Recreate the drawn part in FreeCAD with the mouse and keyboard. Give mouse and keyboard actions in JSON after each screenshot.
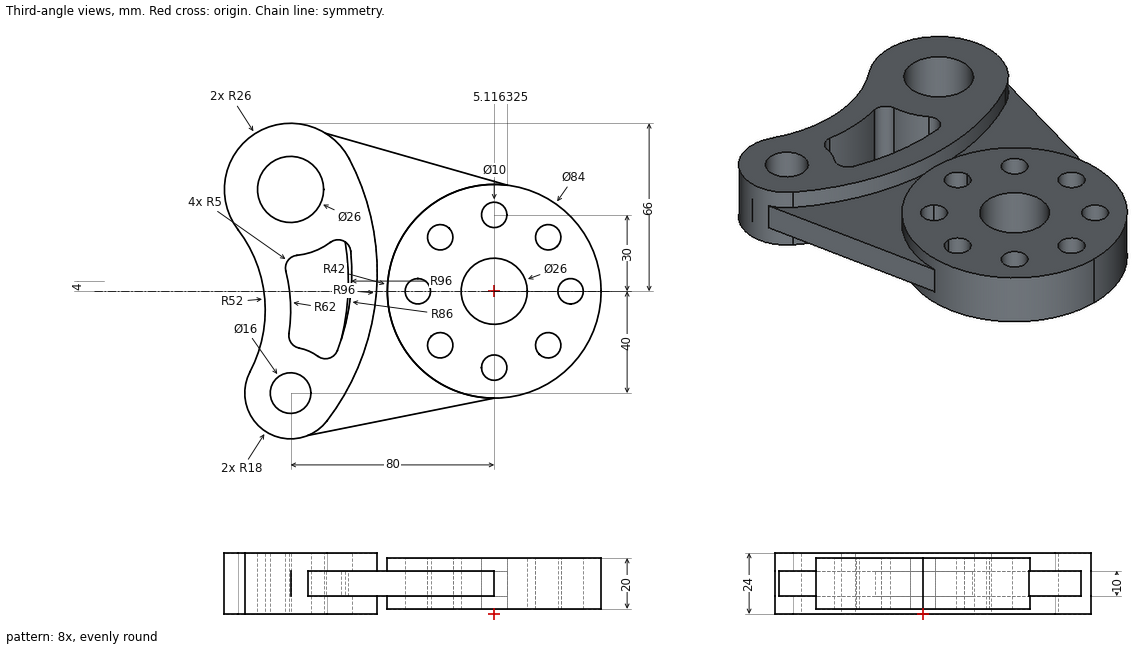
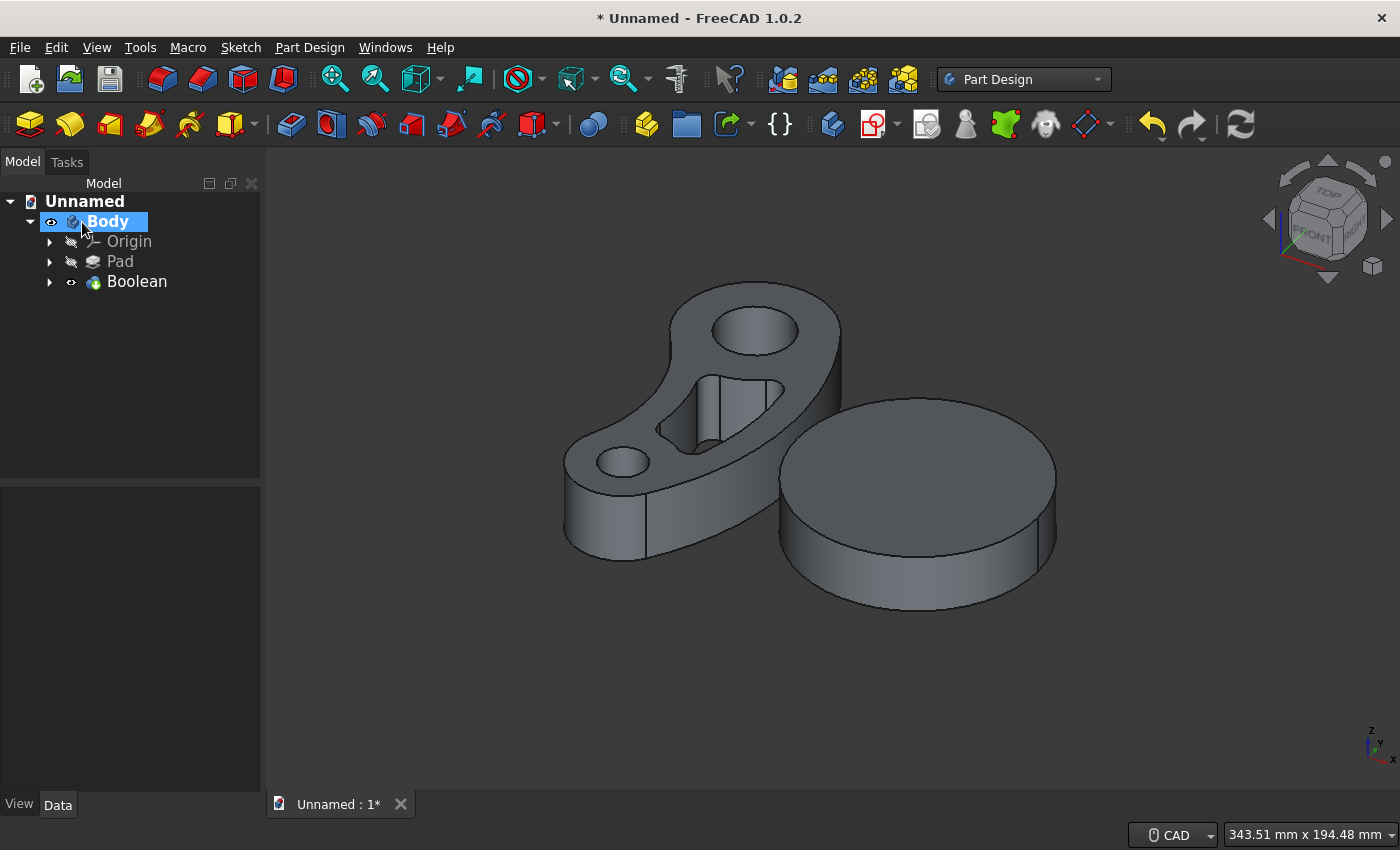
{"action": "left_click", "coordinate": [50, 242]}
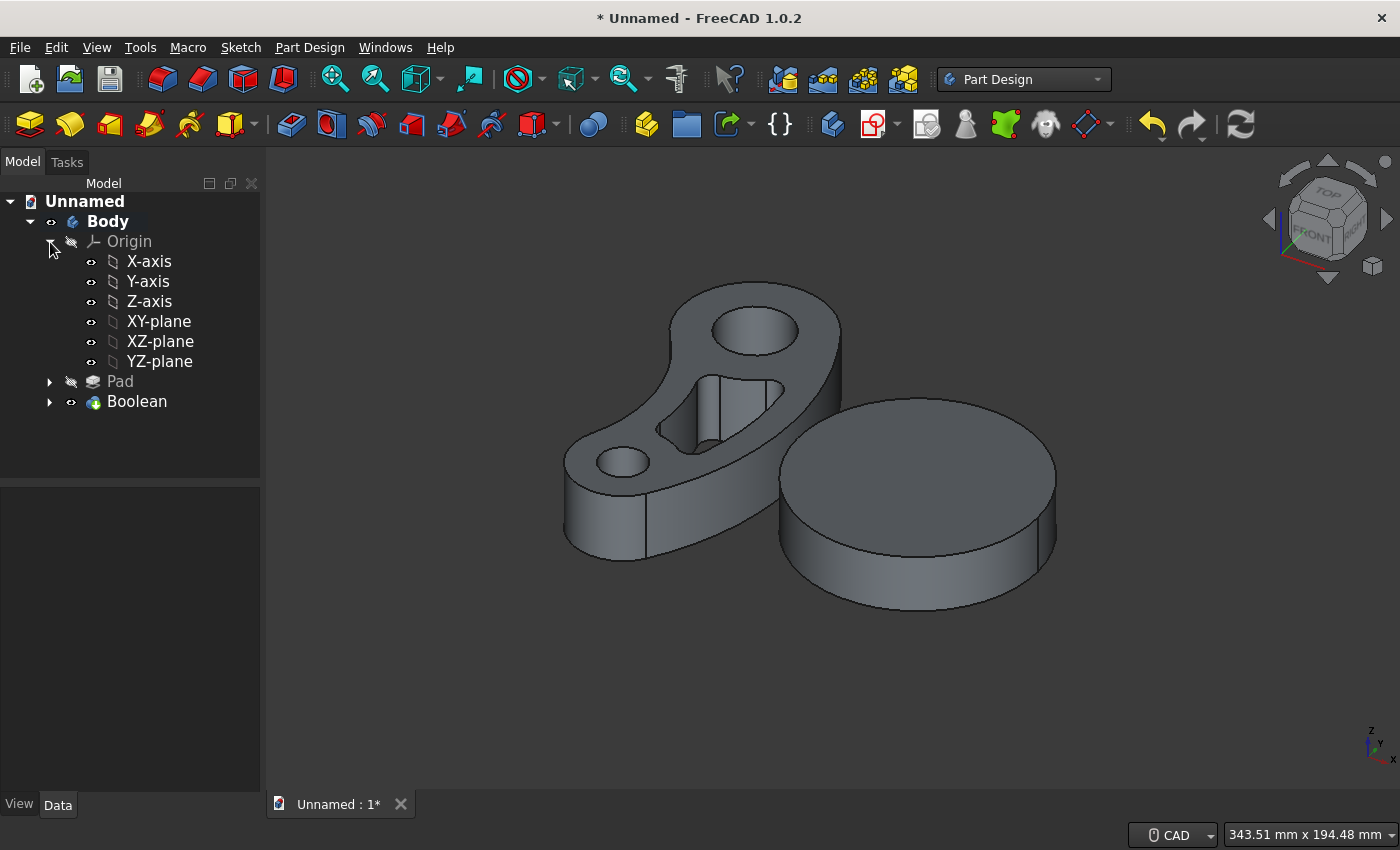
{"action": "left_click", "coordinate": [136, 322]}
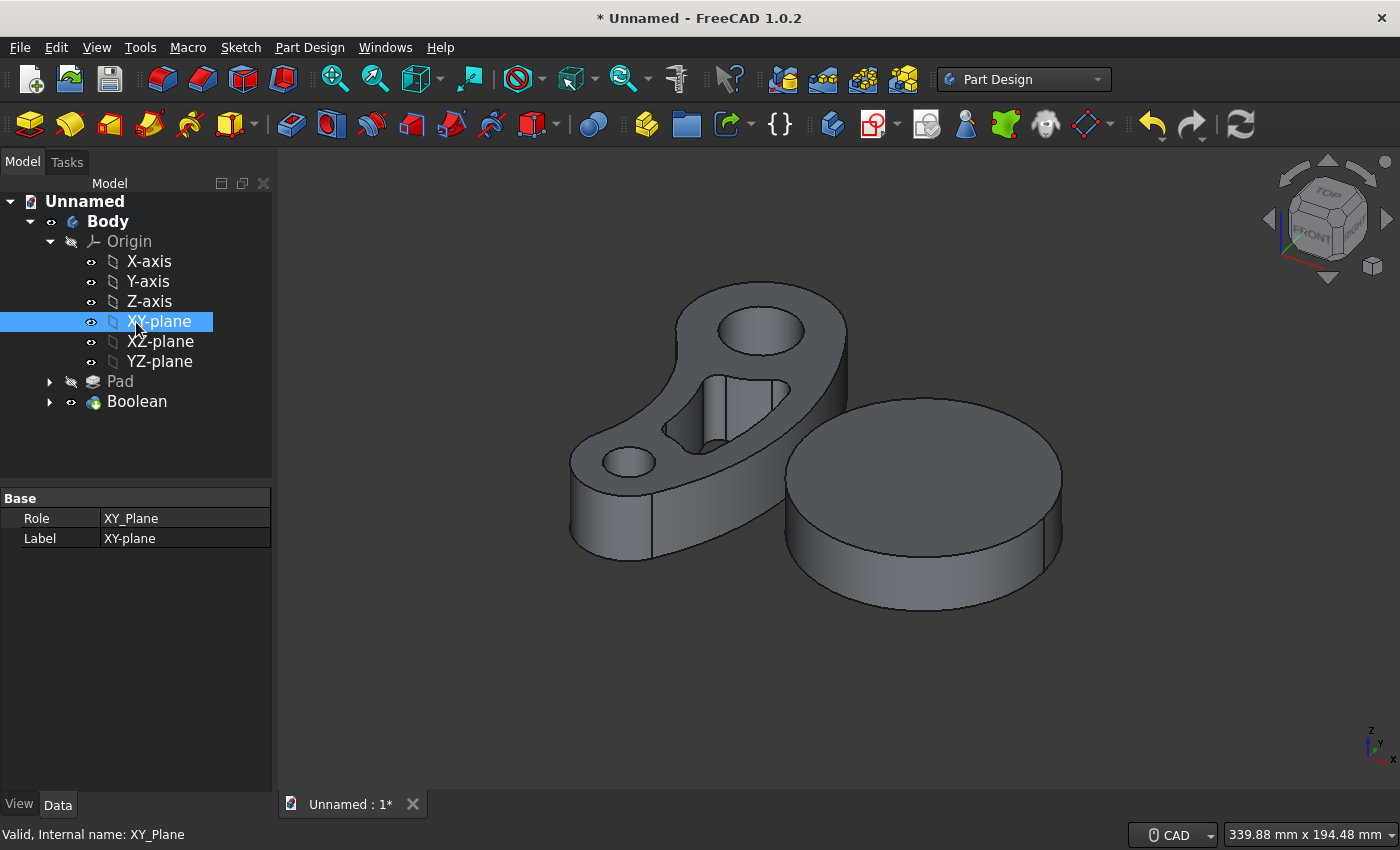
{"action": "left_click", "coordinate": [1086, 124]}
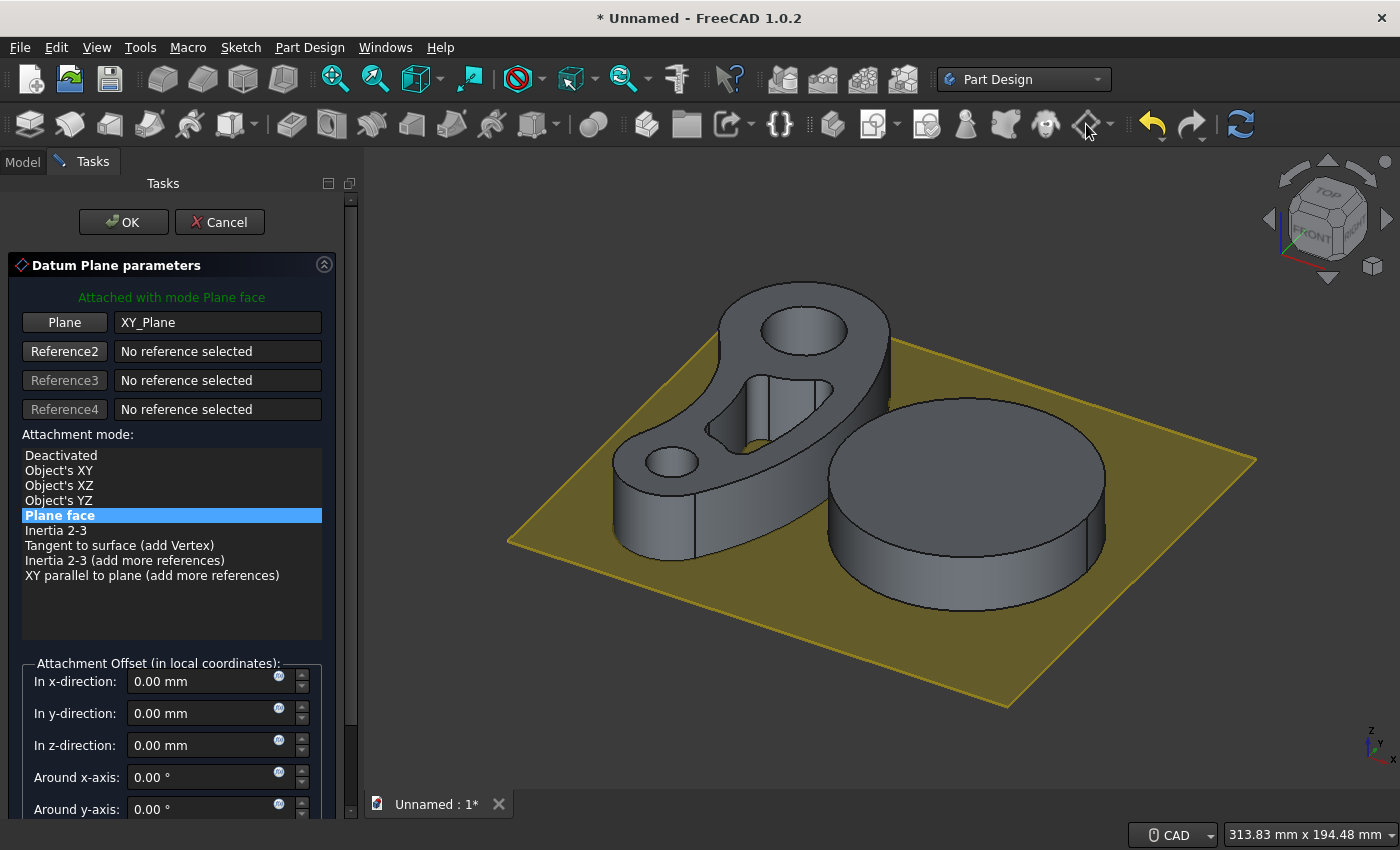
{"action": "triple_click", "coordinate": [210, 745]}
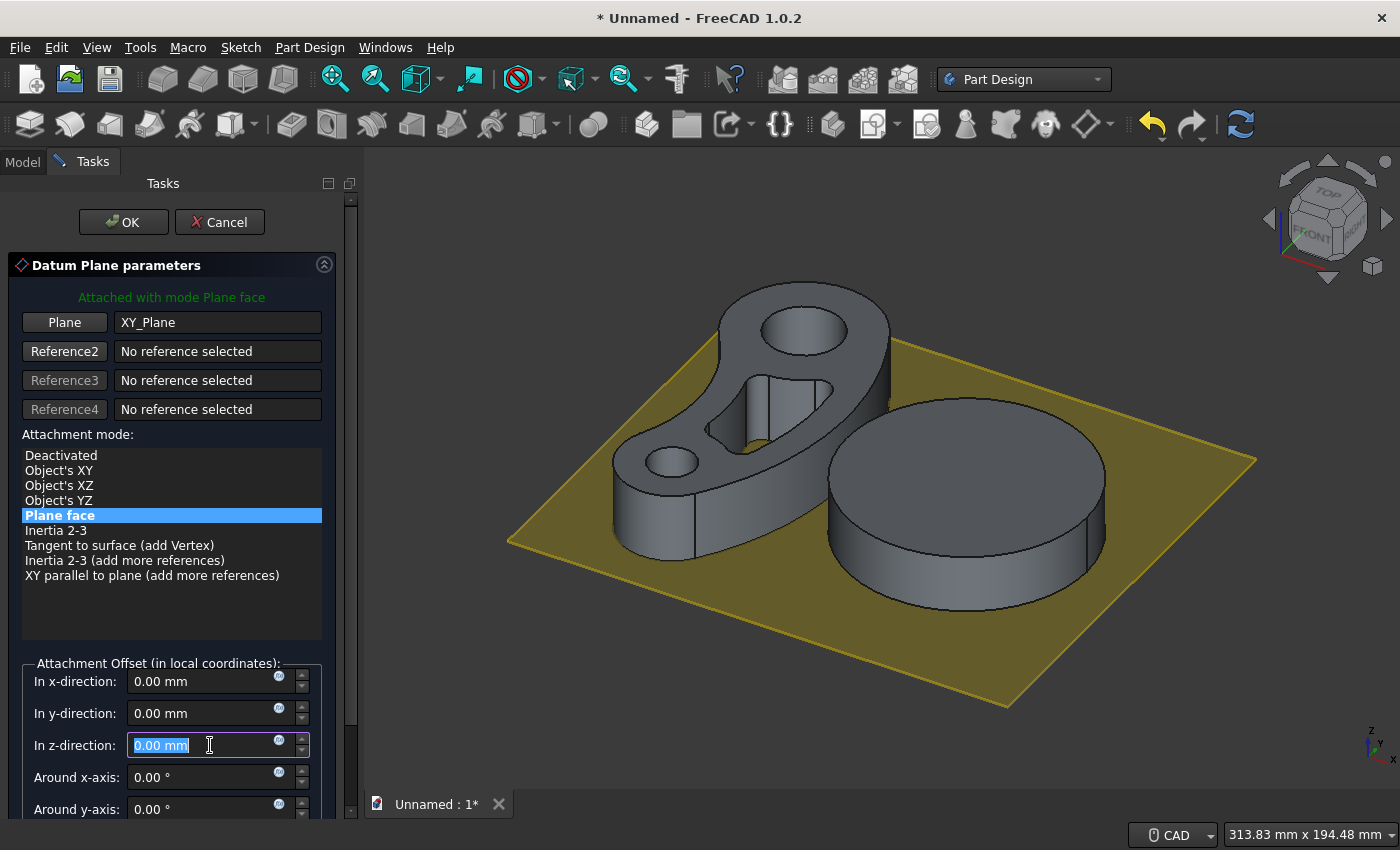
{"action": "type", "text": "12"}
{"action": "key", "text": "Tab"}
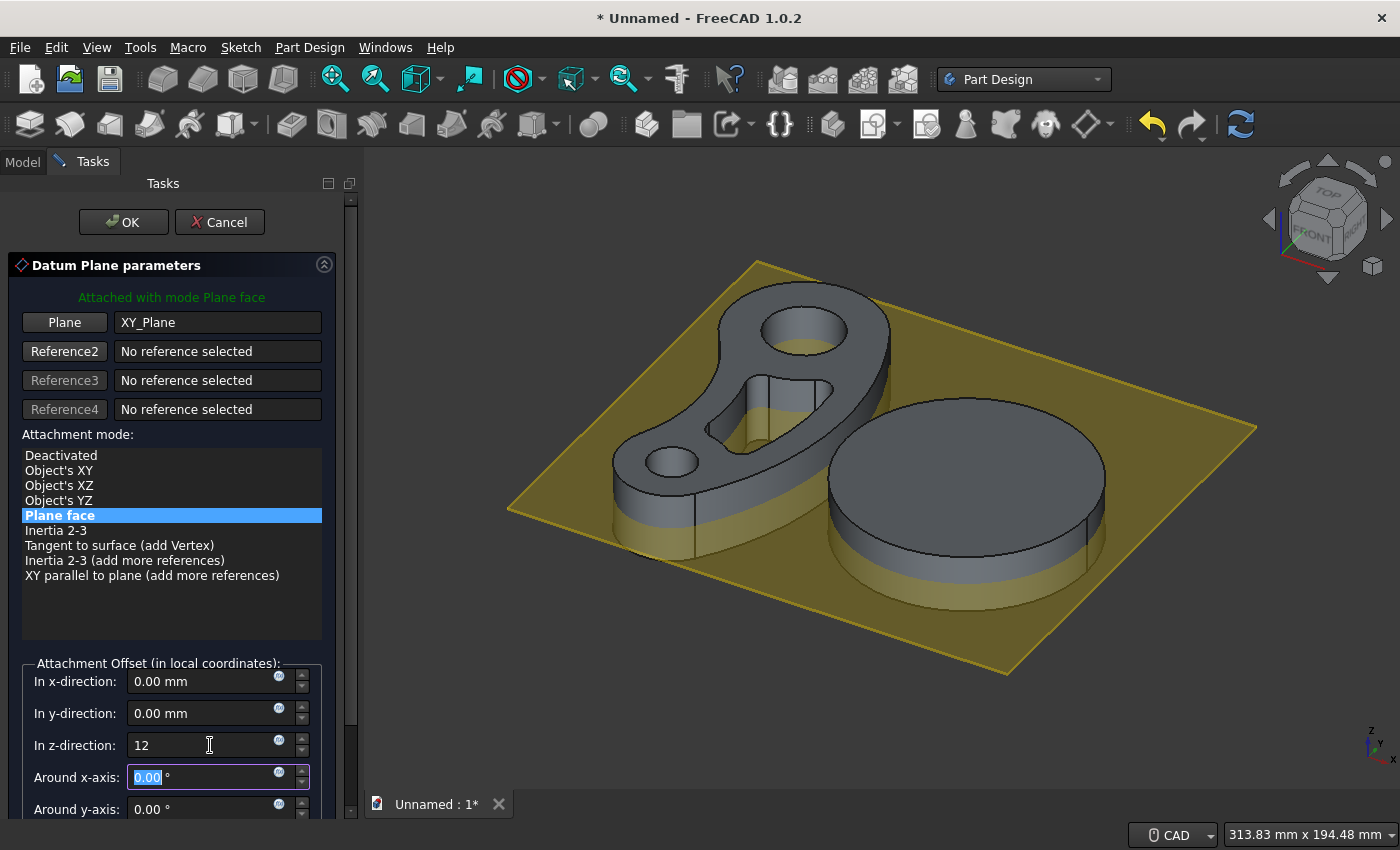
{"action": "left_click", "coordinate": [124, 222]}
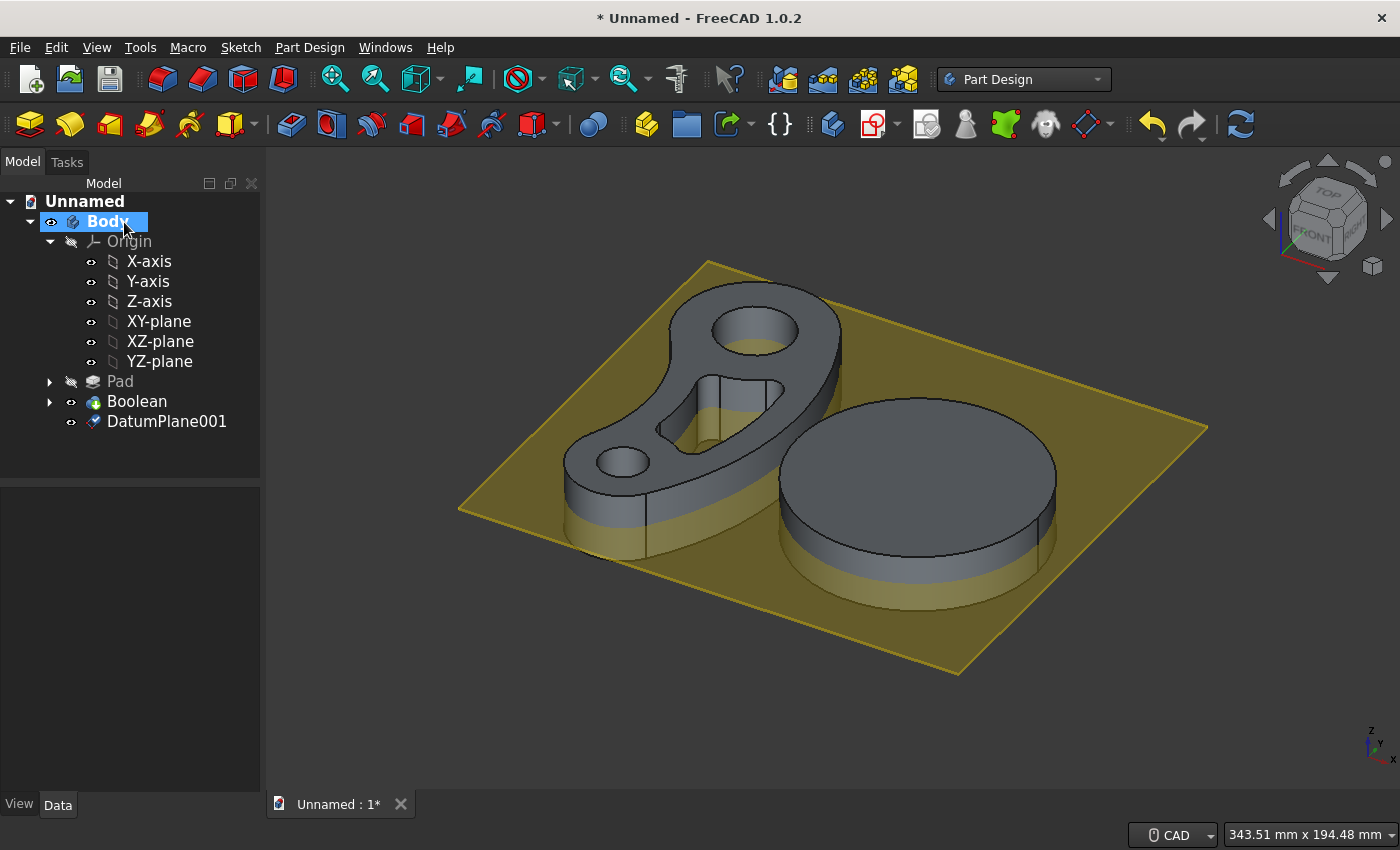
{"action": "left_click", "coordinate": [116, 422]}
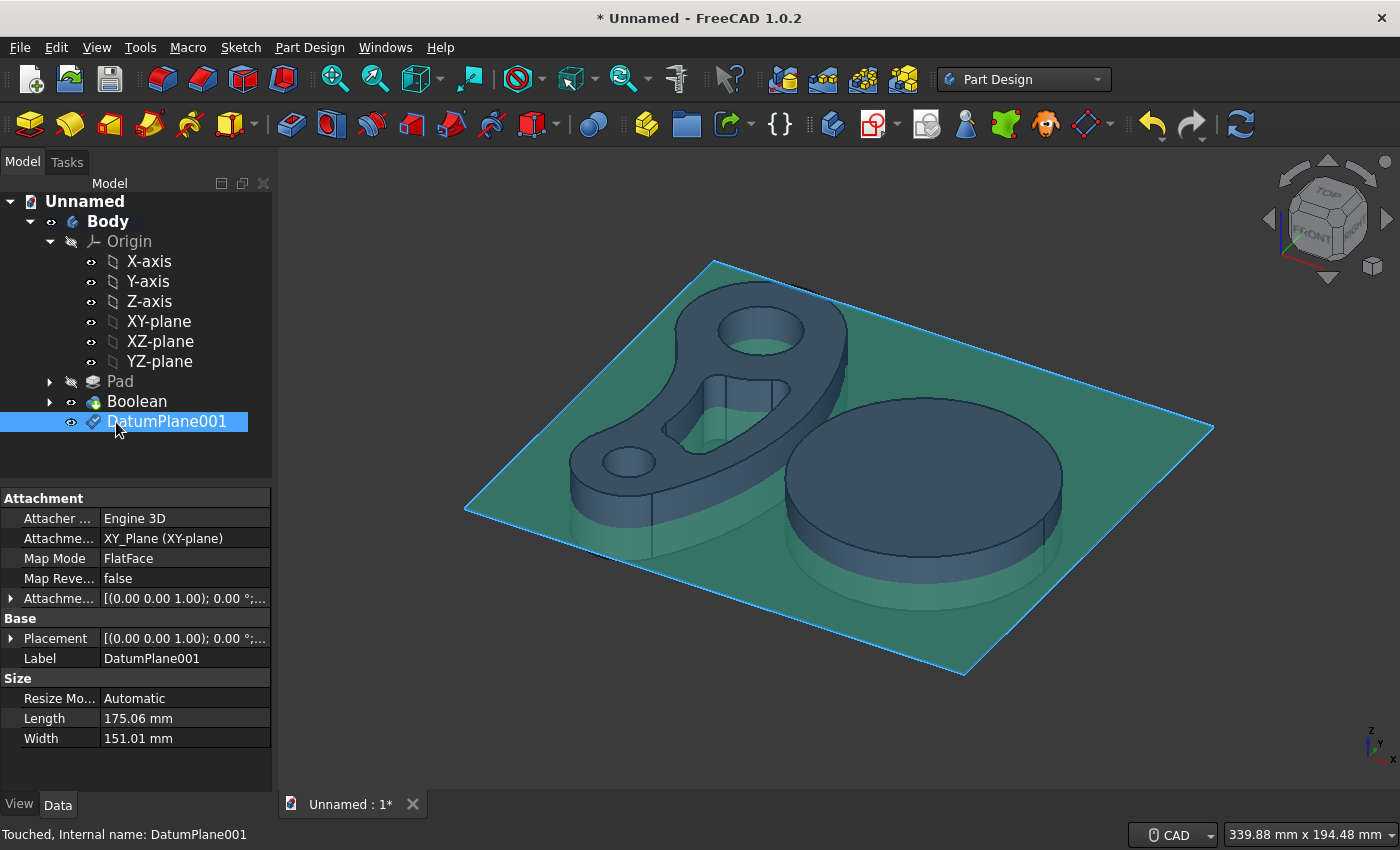
{"action": "left_click", "coordinate": [874, 124]}